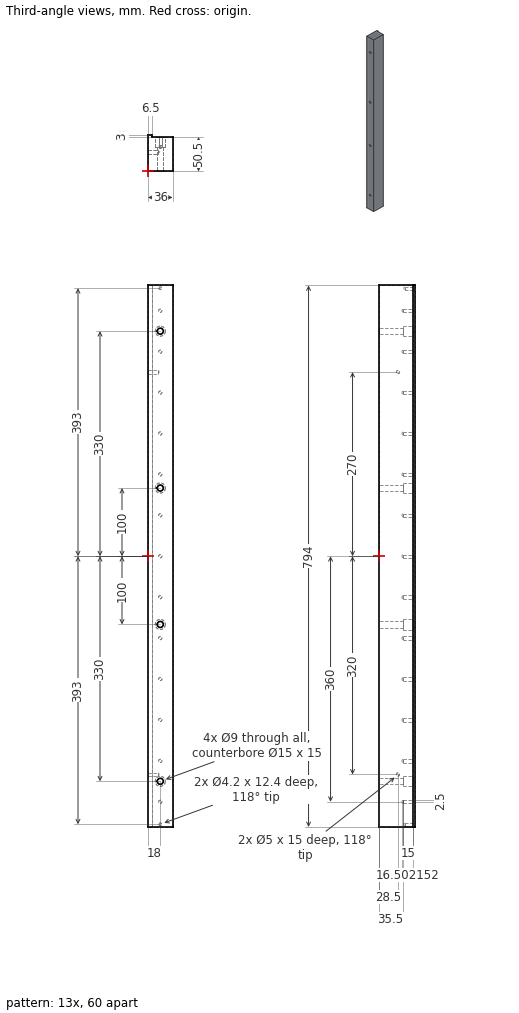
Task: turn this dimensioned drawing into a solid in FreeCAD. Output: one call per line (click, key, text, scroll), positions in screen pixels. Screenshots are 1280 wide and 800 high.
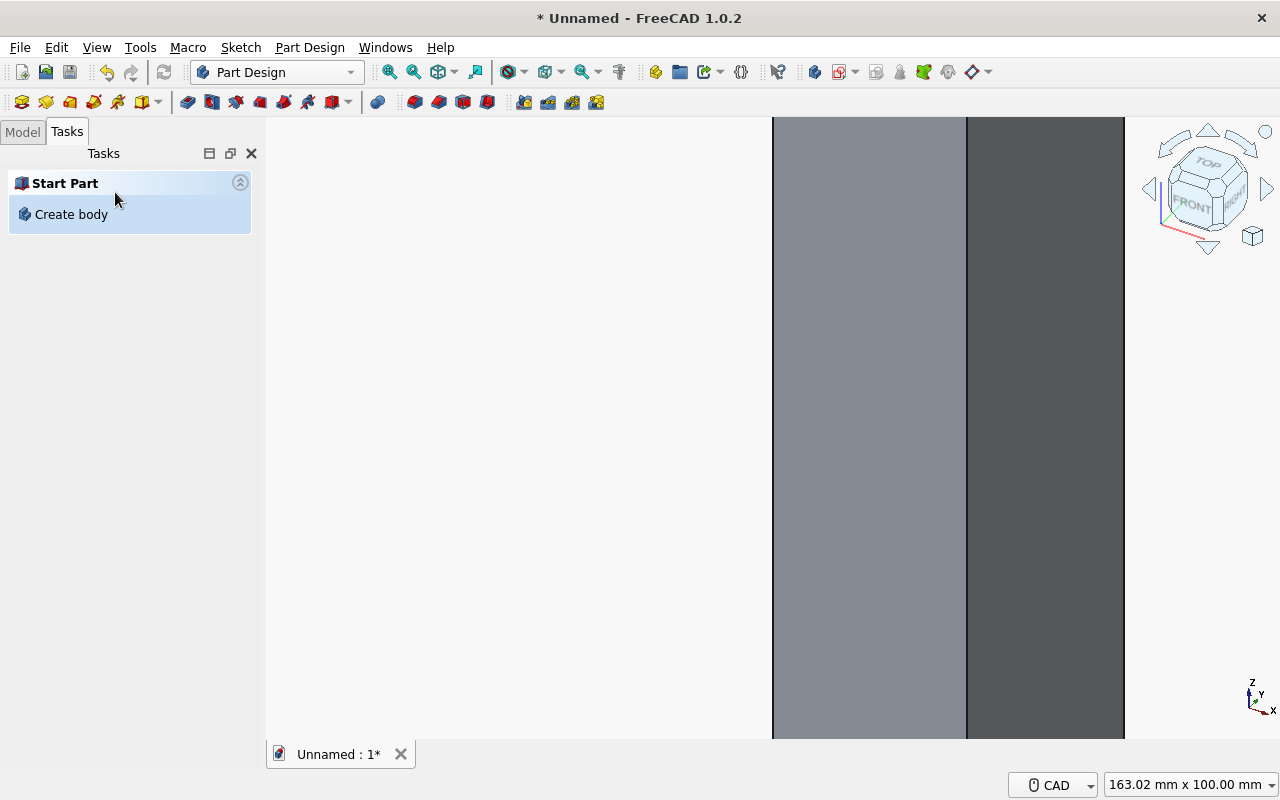
click(390, 72)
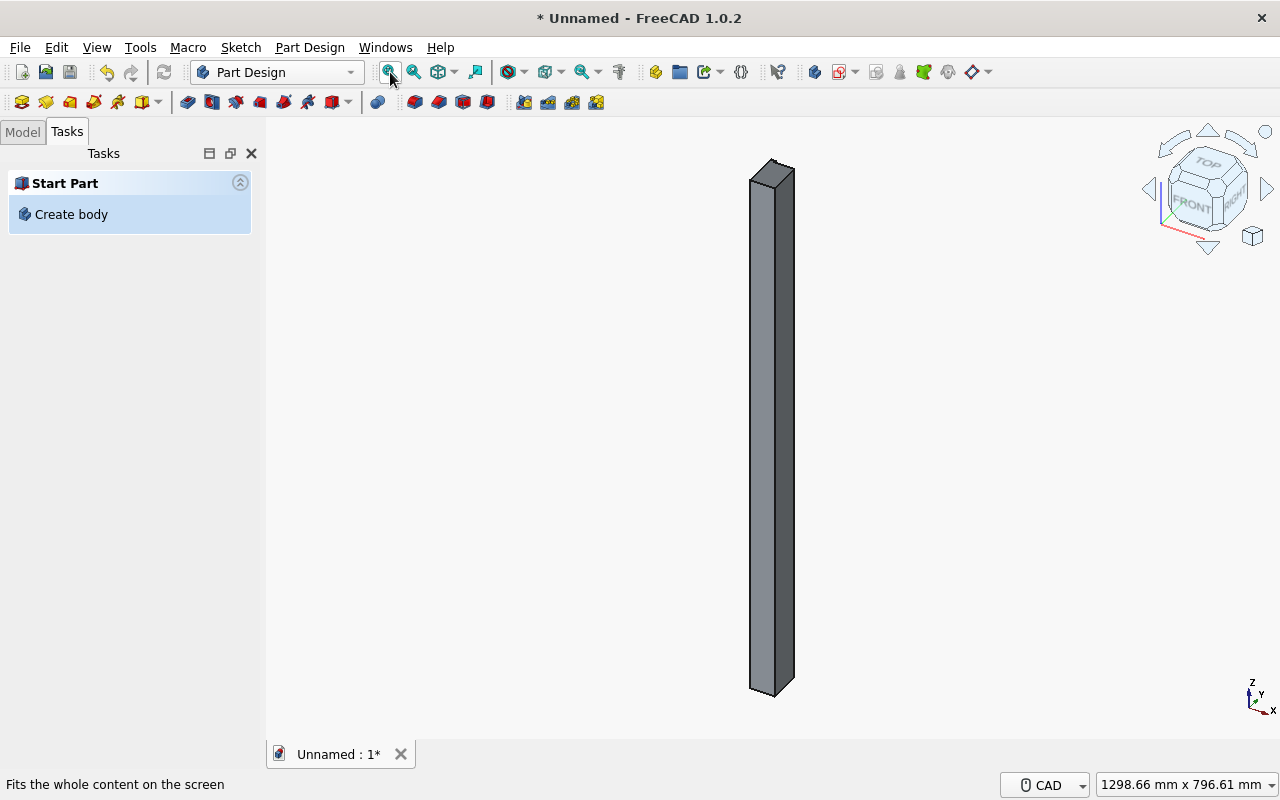
click(840, 72)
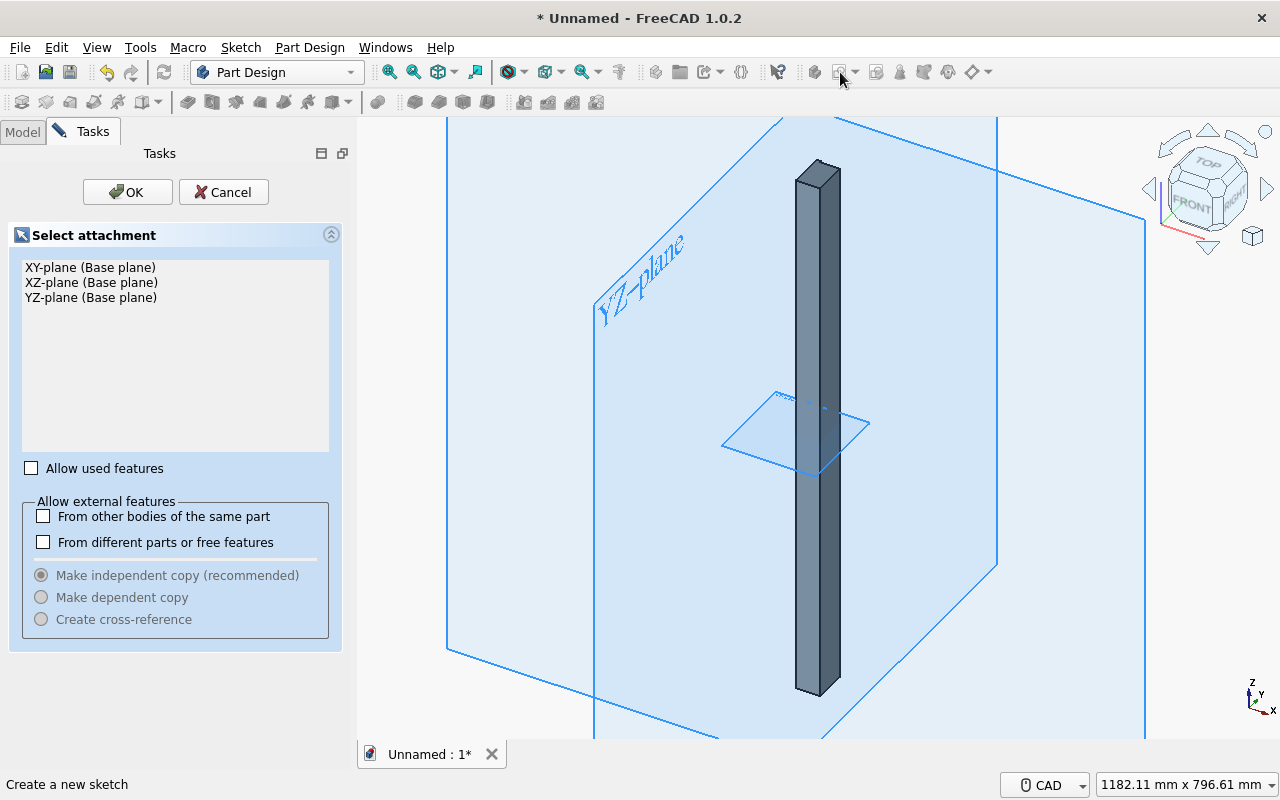
click(82, 298)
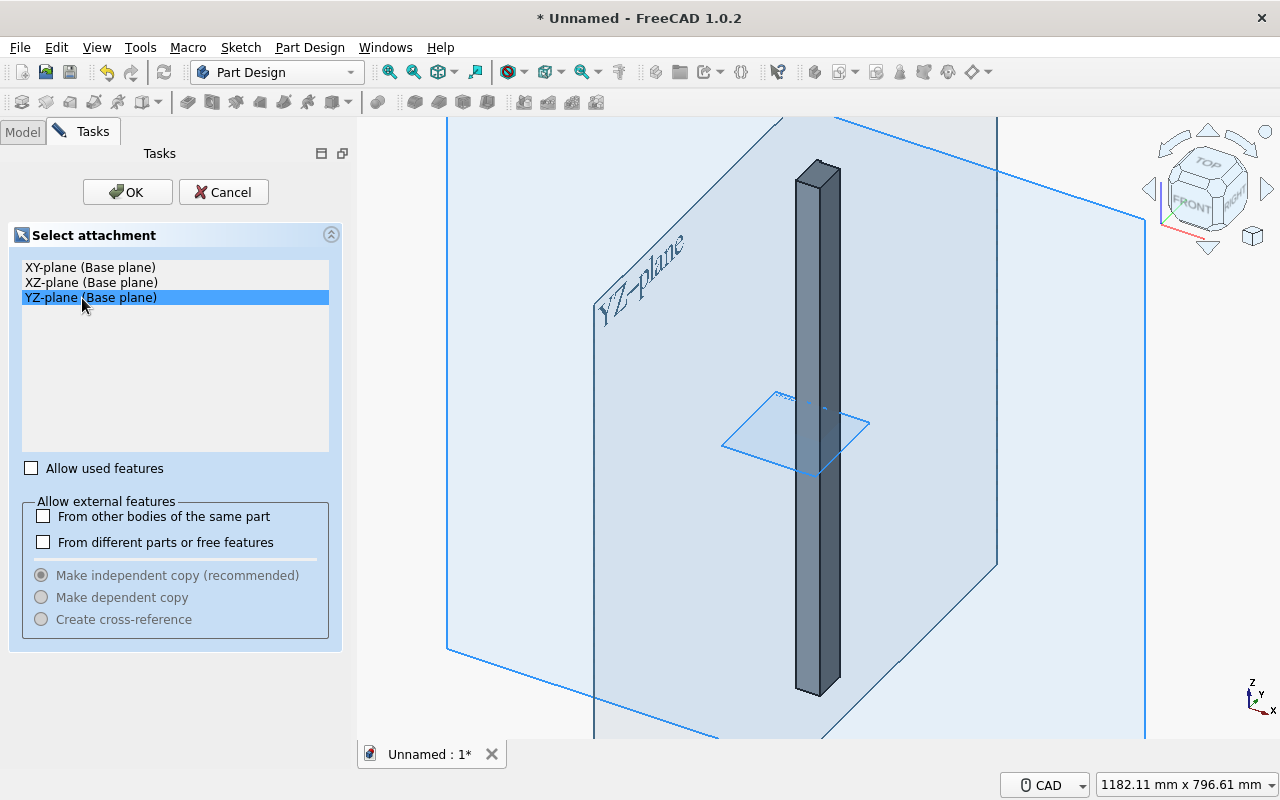
click(128, 192)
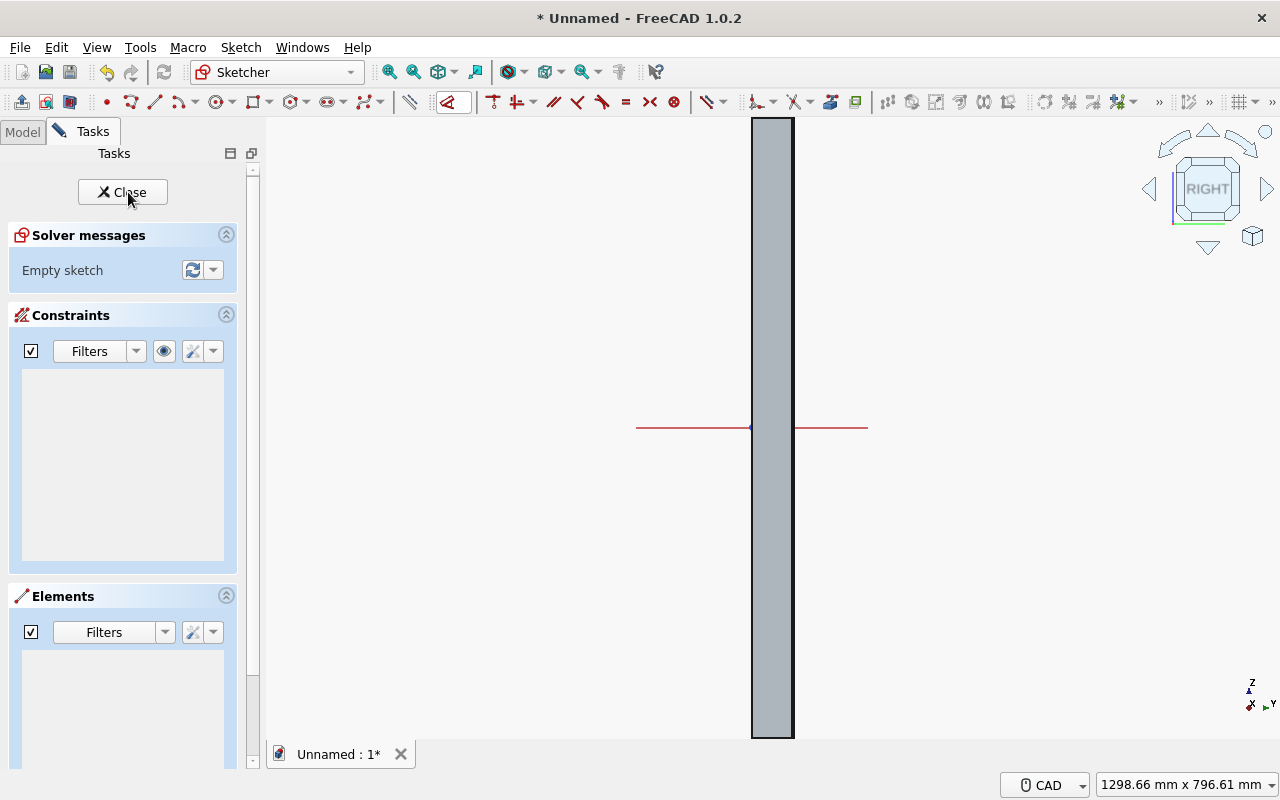
click(70, 102)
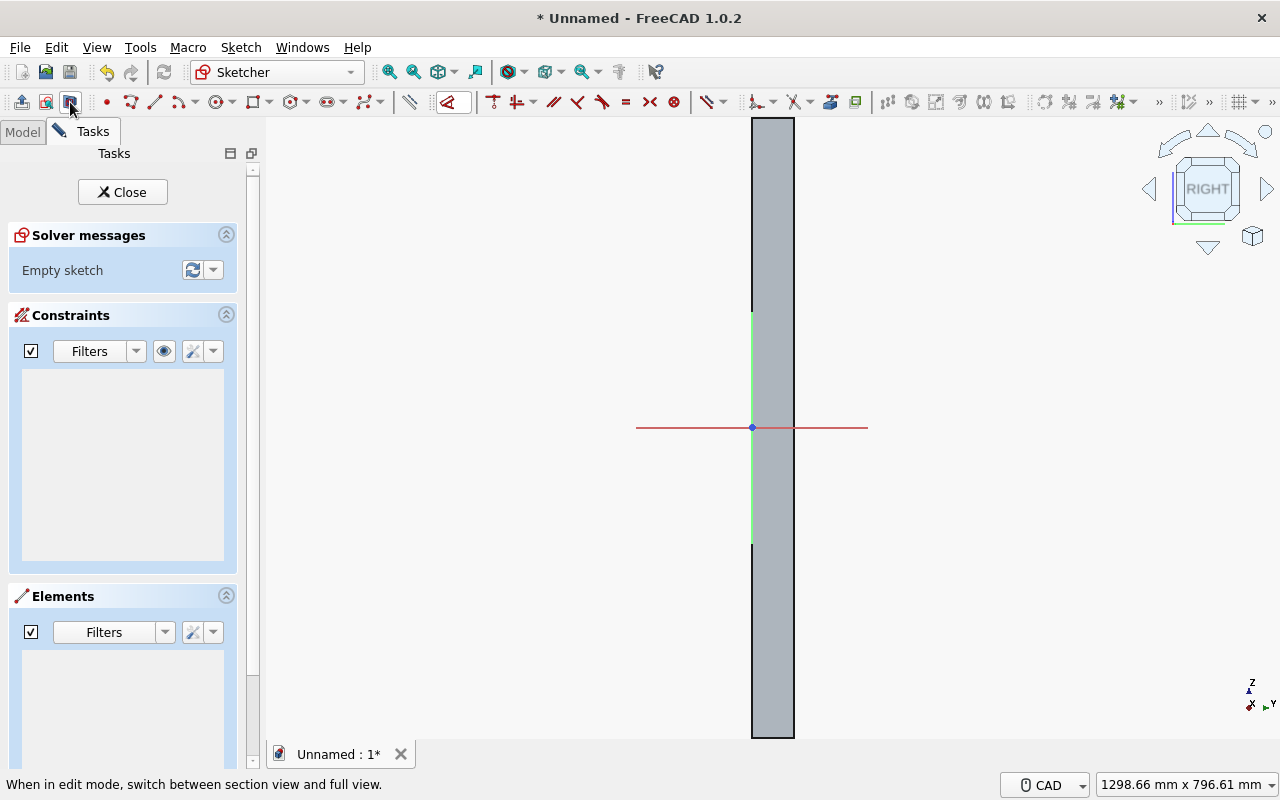
click(216, 102)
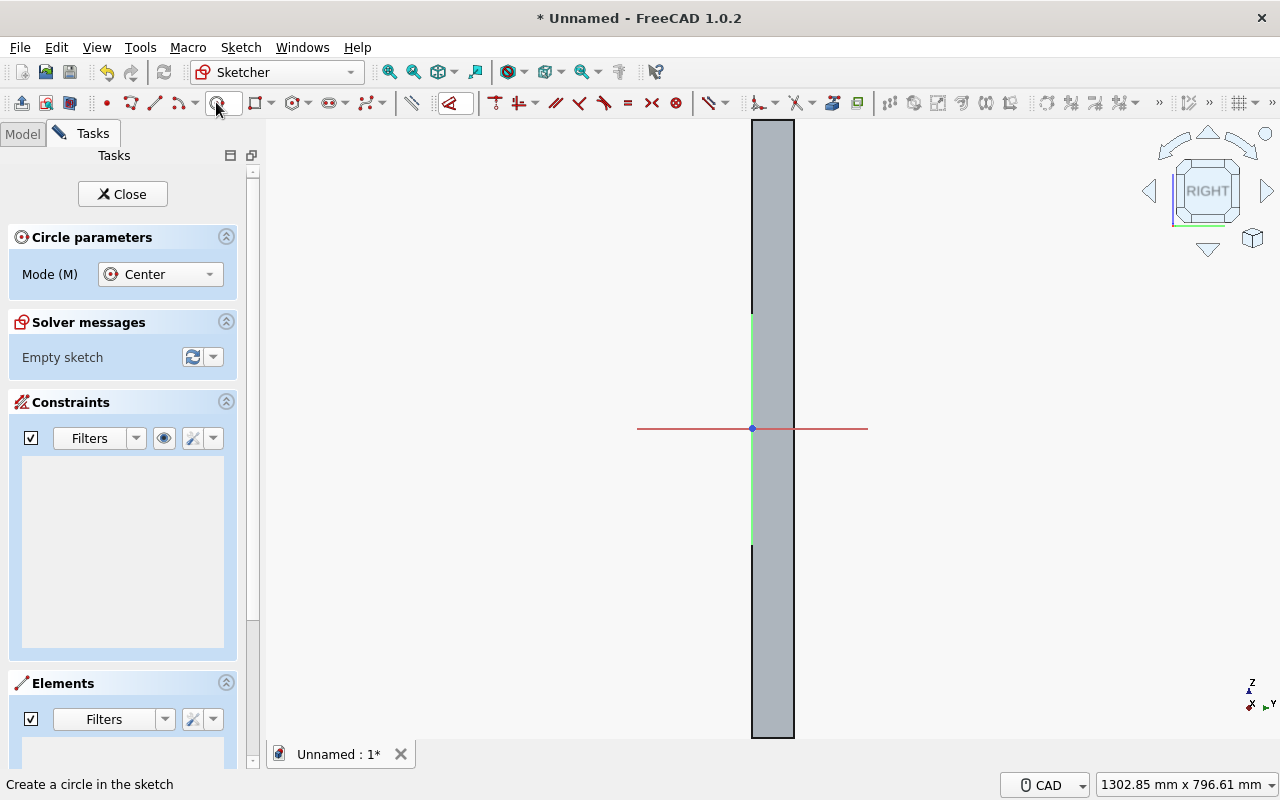
scroll(774, 678, up, 13)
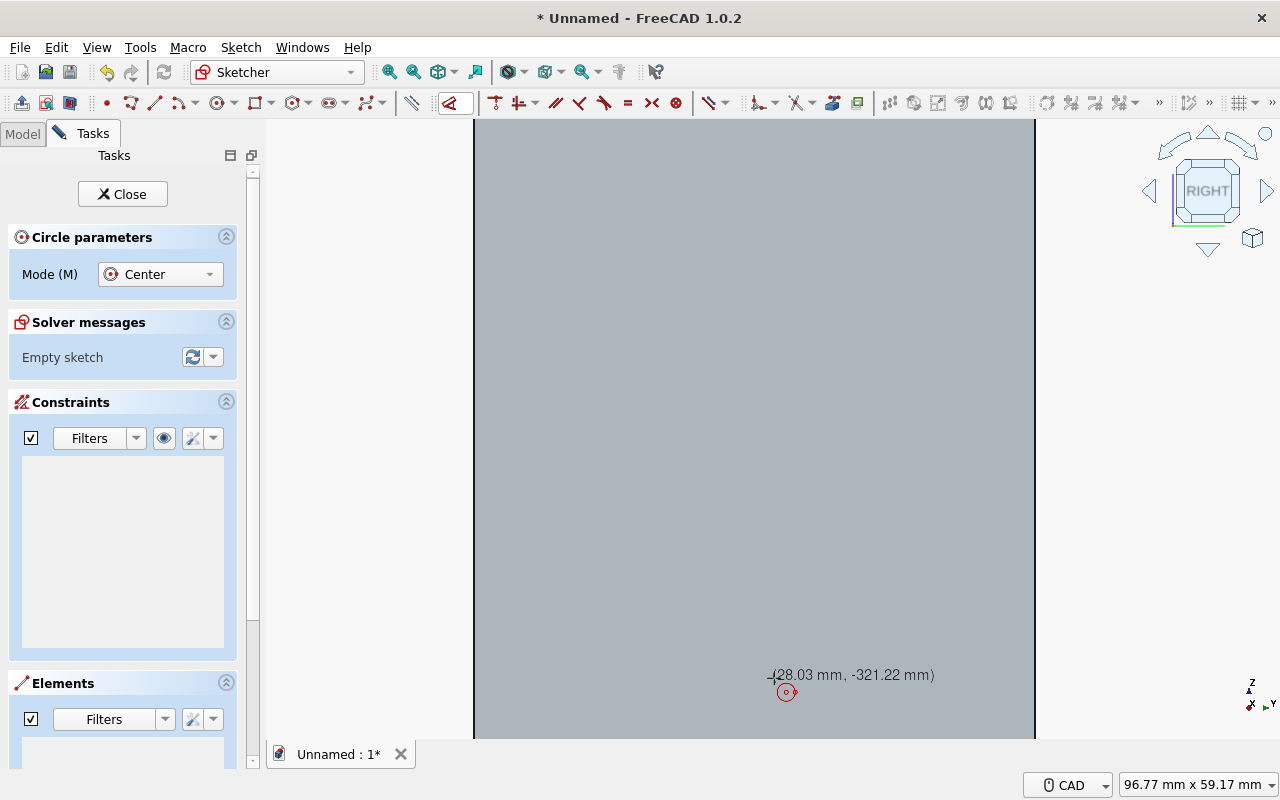
scroll(709, 614, down, 14)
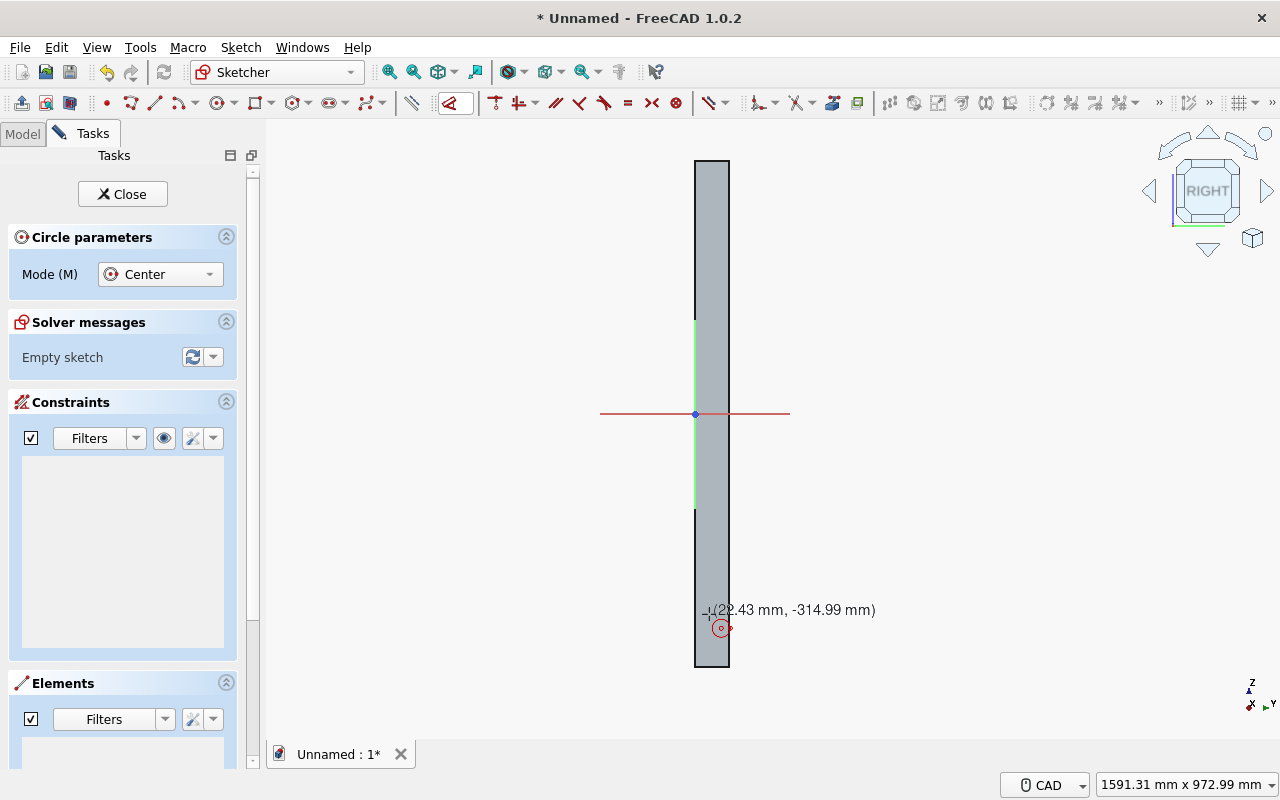
click(713, 618)
move(714, 617)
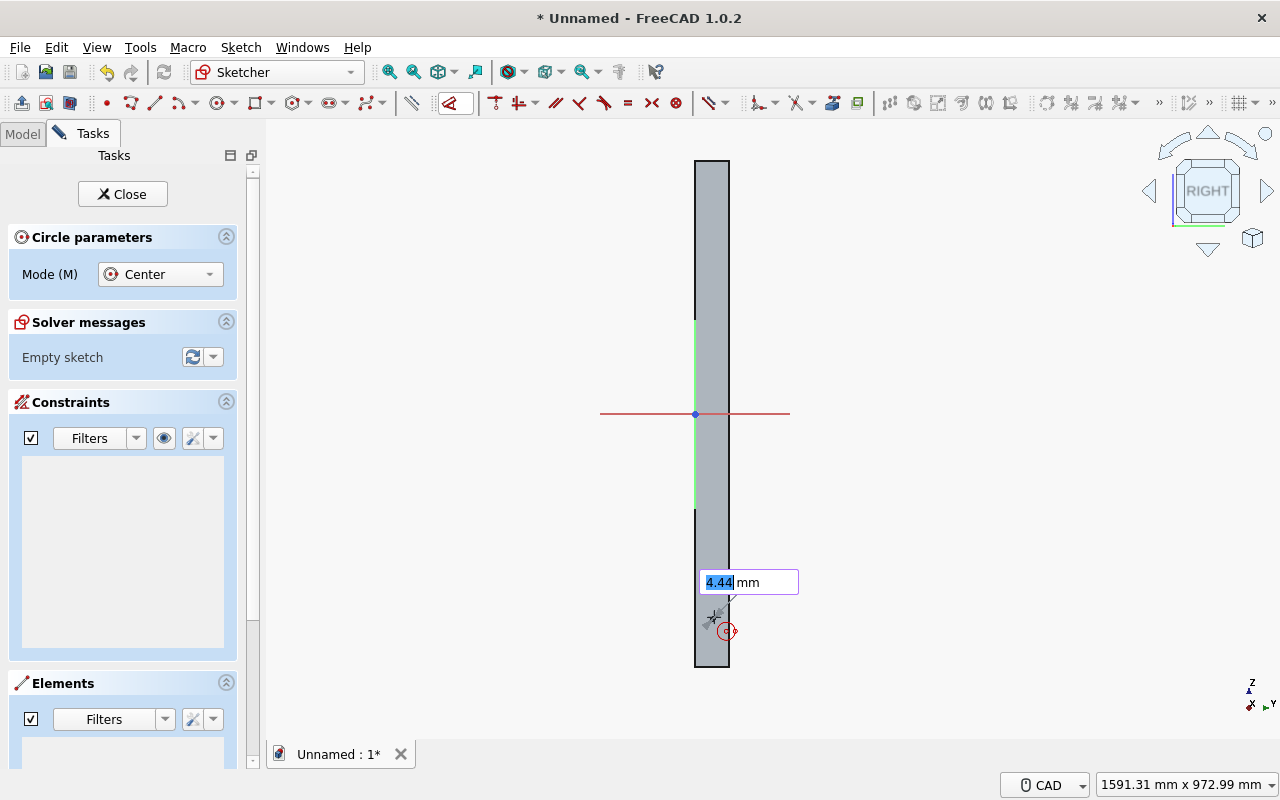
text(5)
key(Return)